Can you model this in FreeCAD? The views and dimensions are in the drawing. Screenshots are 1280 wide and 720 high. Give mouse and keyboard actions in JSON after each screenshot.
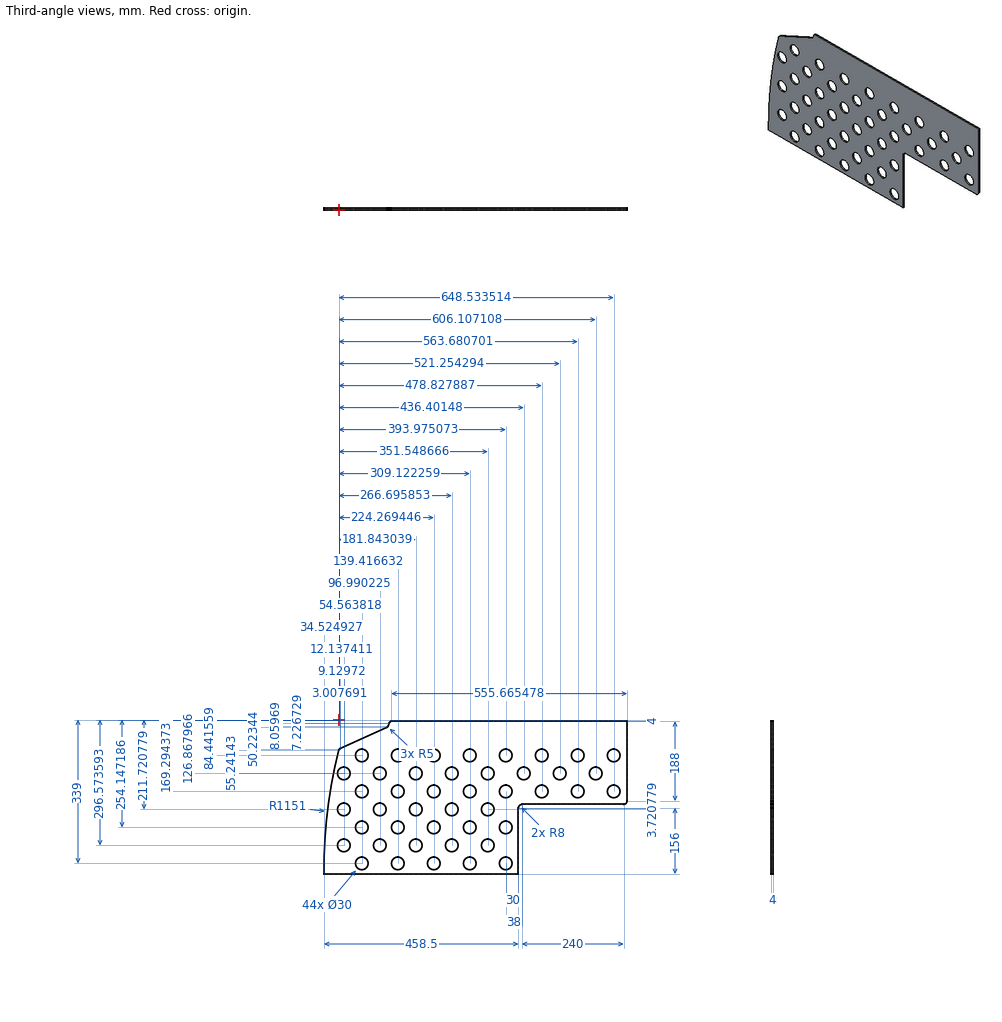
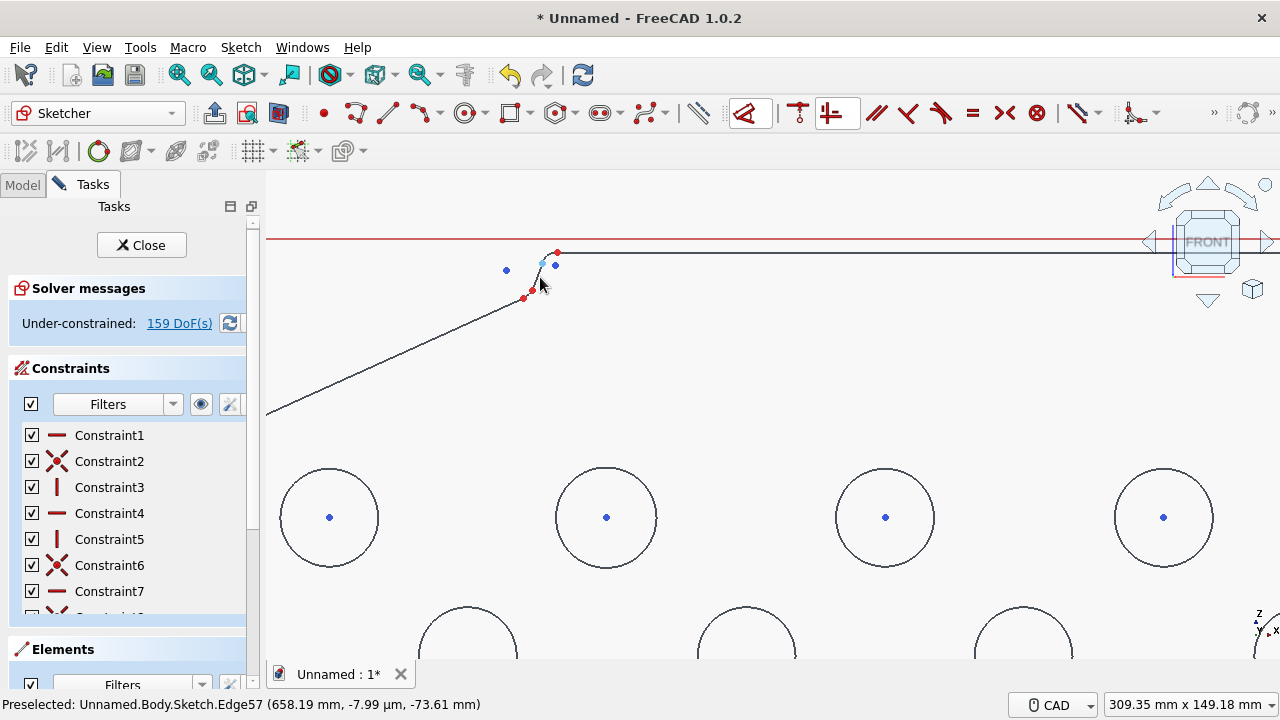
{"action": "left_click", "coordinate": [537, 277]}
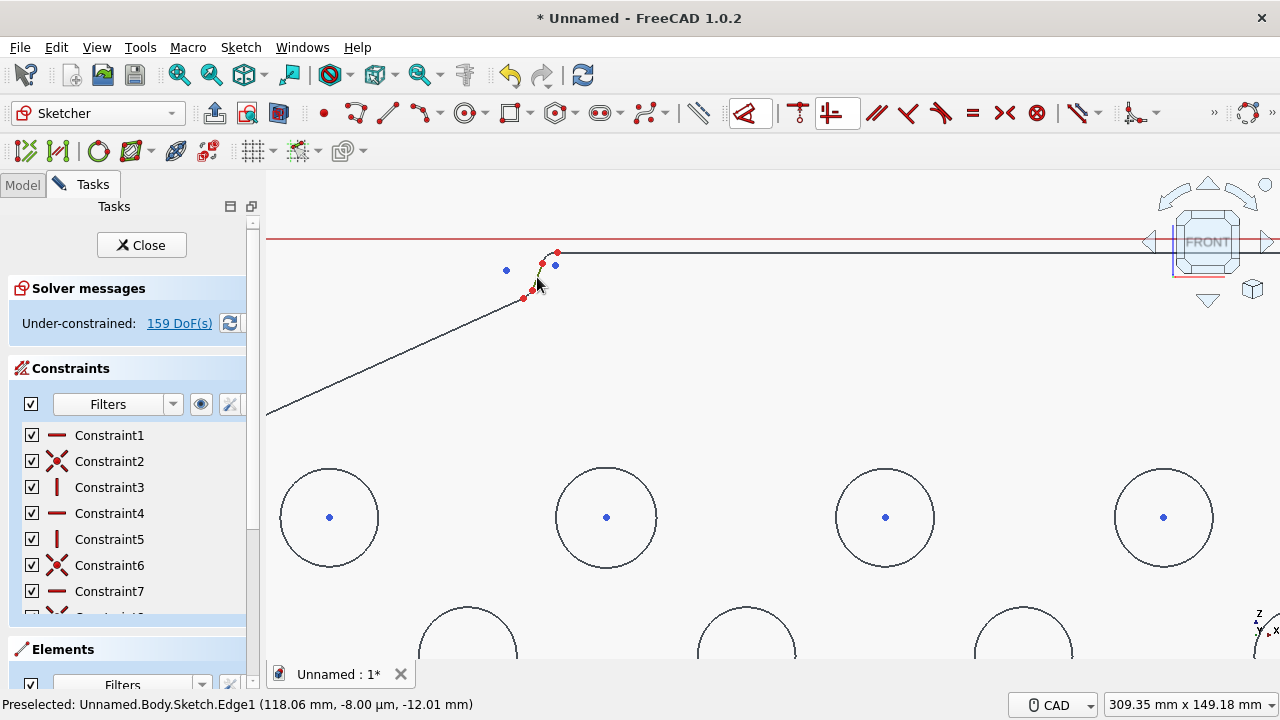
{"action": "scroll", "coordinate": [528, 295], "scroll_direction": "up", "scroll_amount": 5}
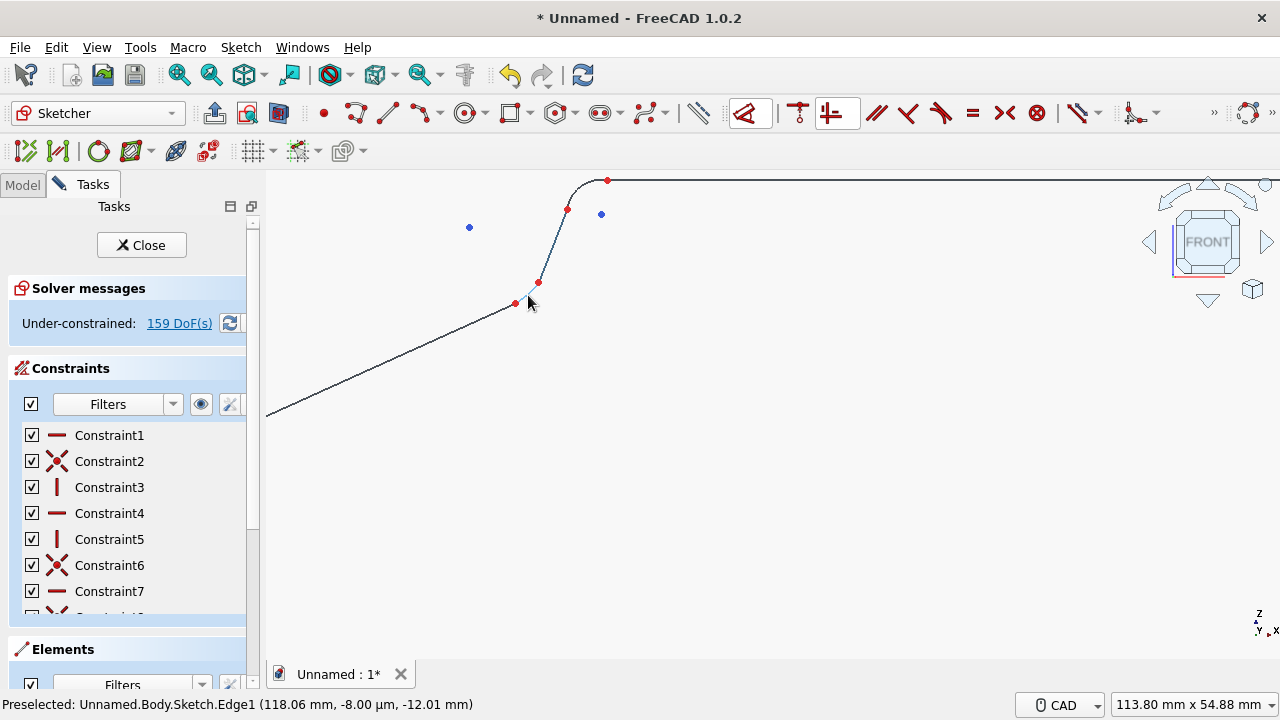
{"action": "left_click", "coordinate": [528, 294]}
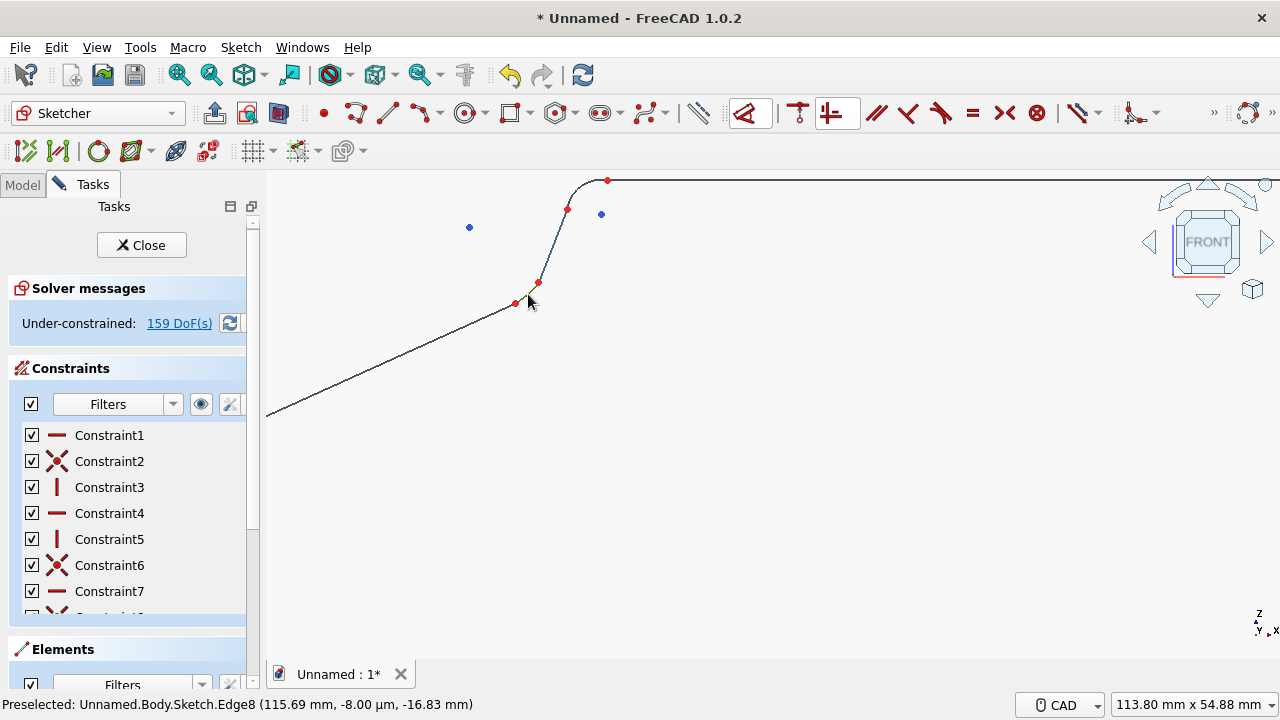
{"action": "key", "text": "t"}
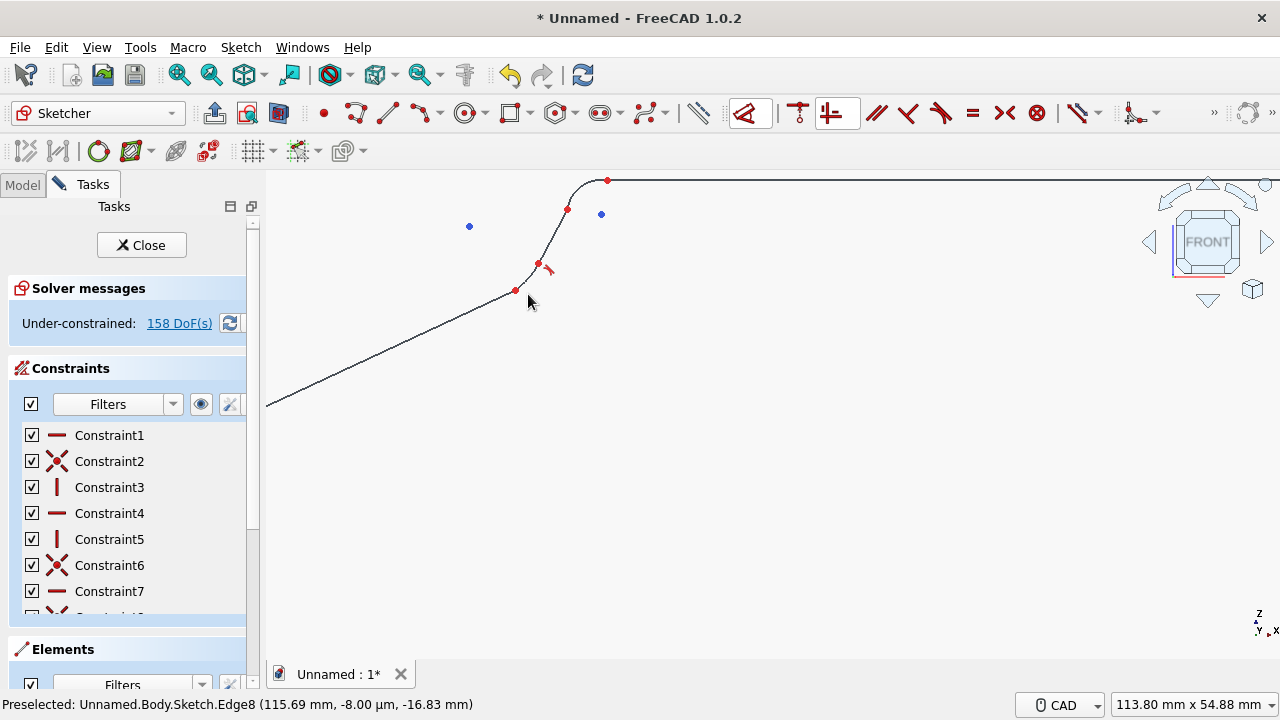
{"action": "left_click", "coordinate": [559, 226]}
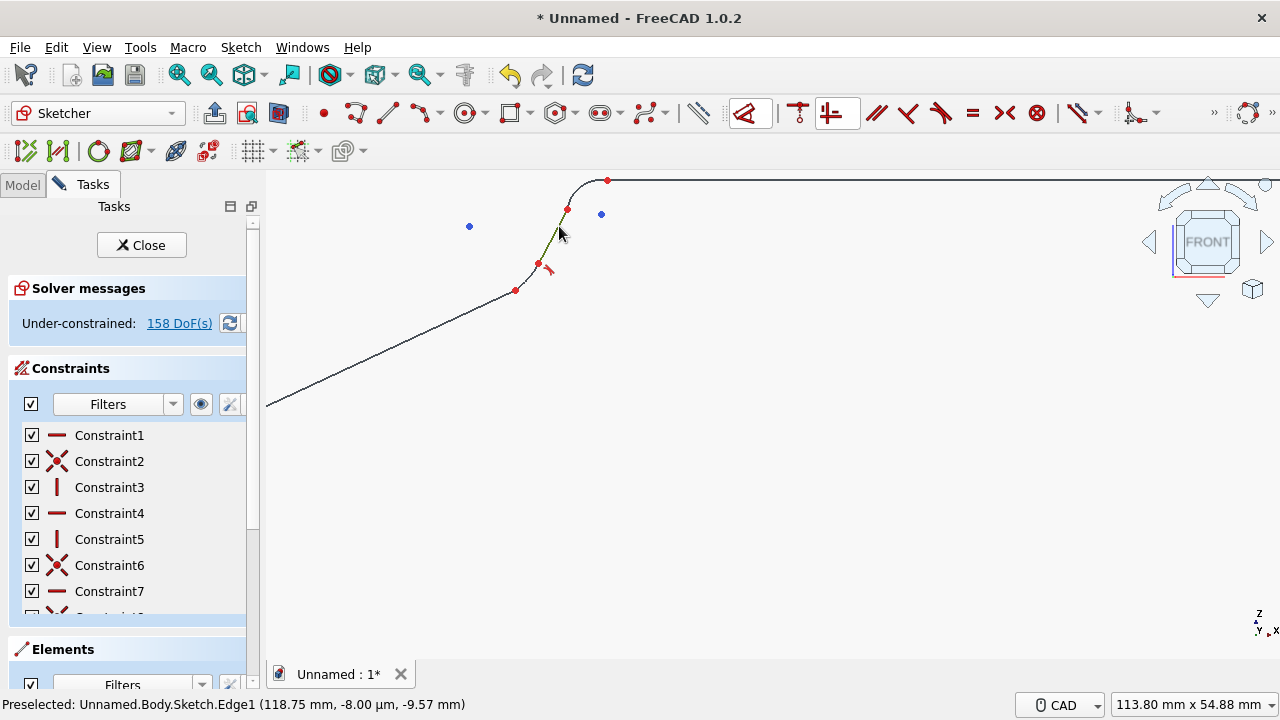
{"action": "scroll", "coordinate": [571, 199], "scroll_direction": "up", "scroll_amount": 2}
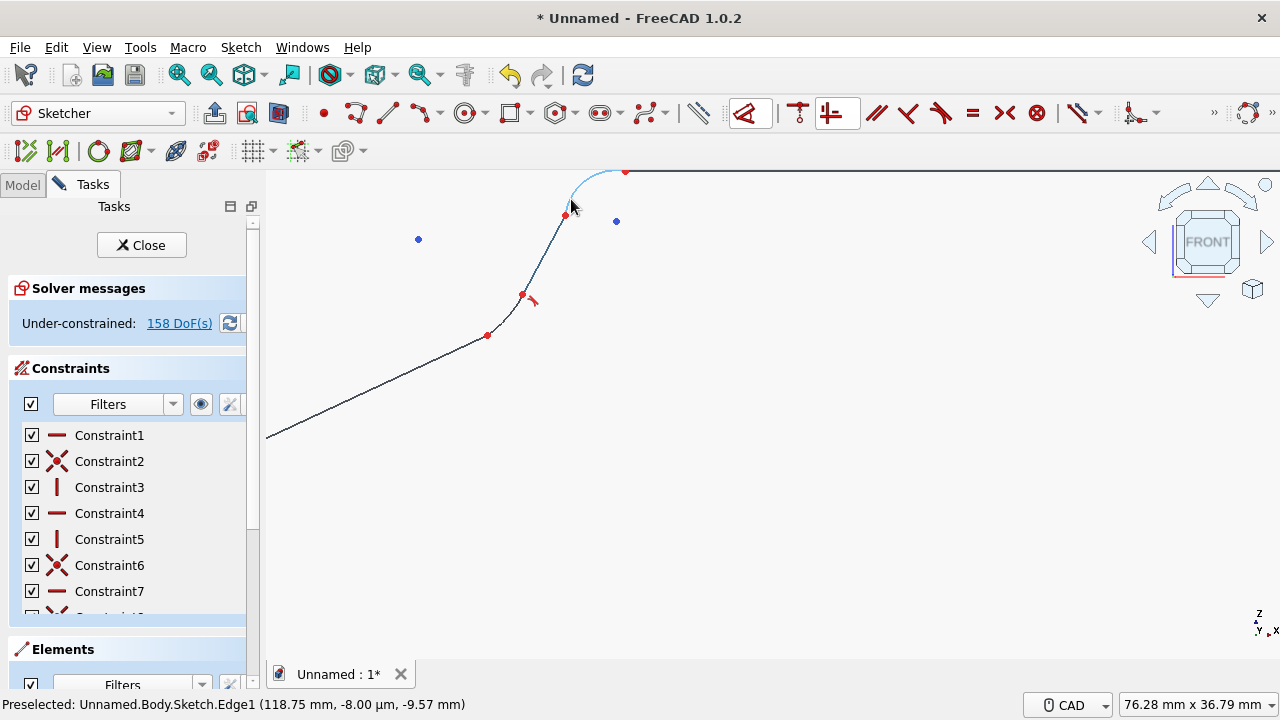
{"action": "left_click", "coordinate": [570, 199]}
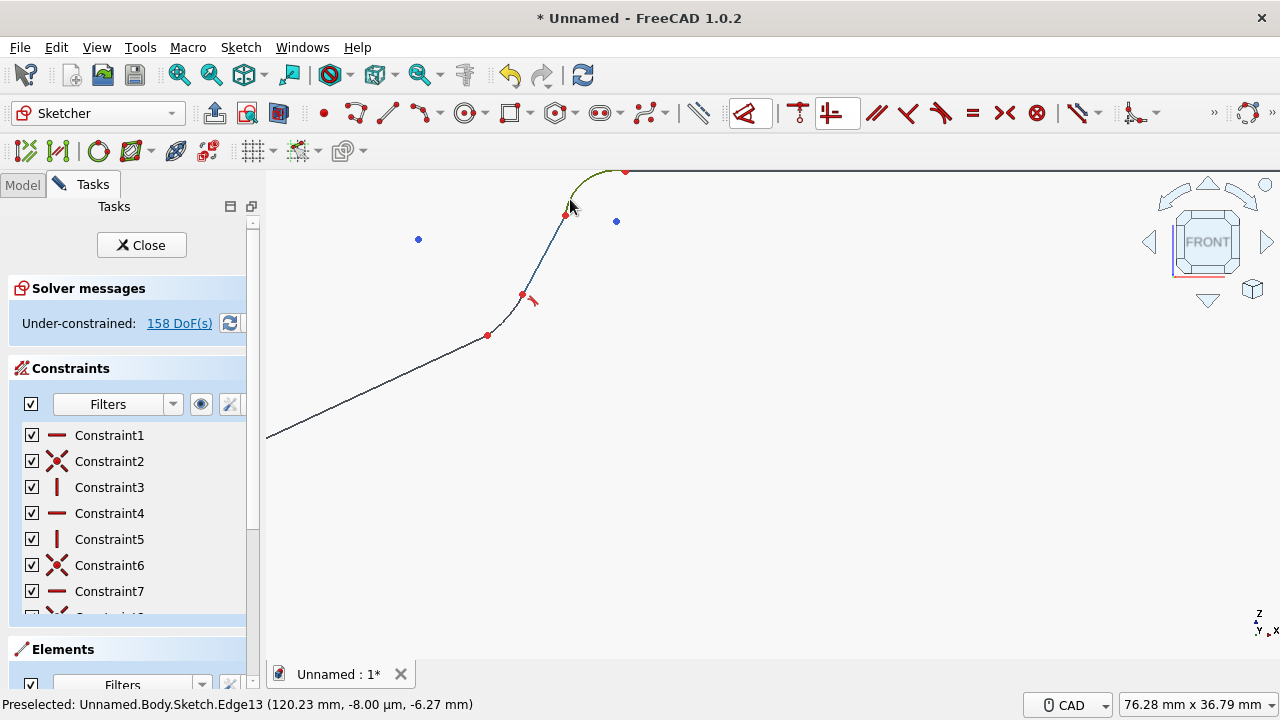
{"action": "left_click", "coordinate": [942, 114]}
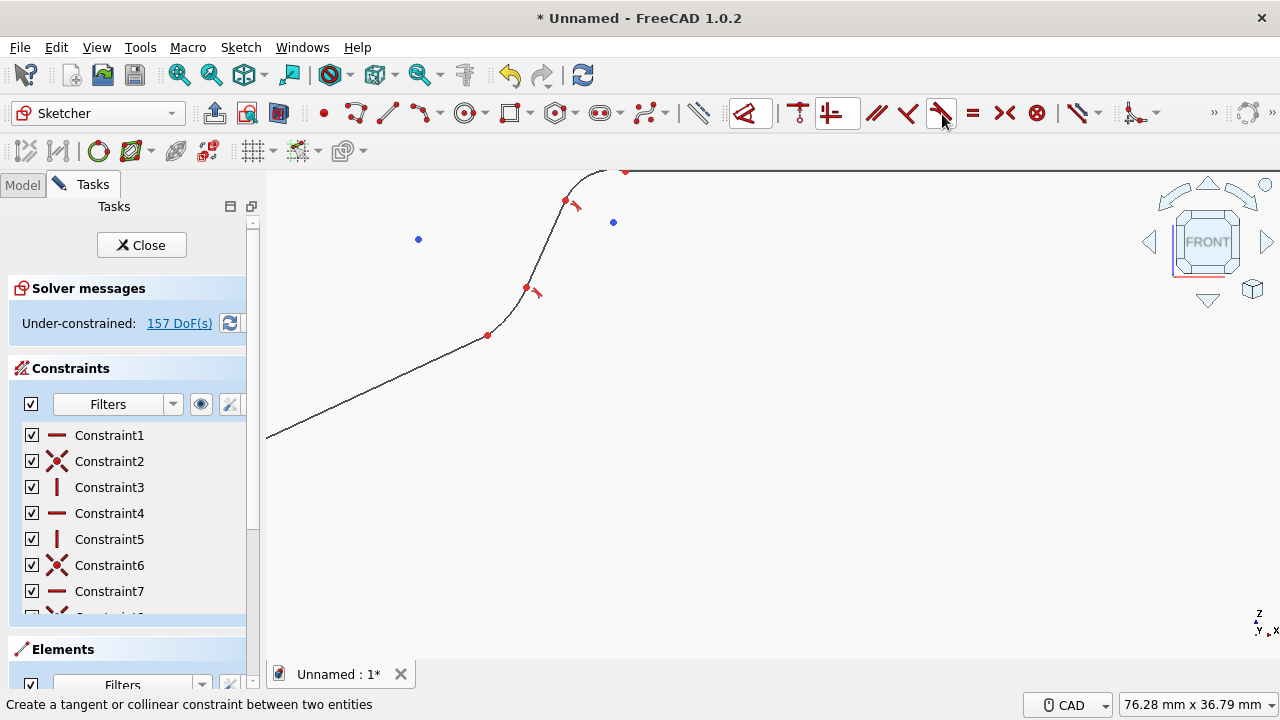
{"action": "scroll", "coordinate": [539, 277], "scroll_direction": "down", "scroll_amount": 14}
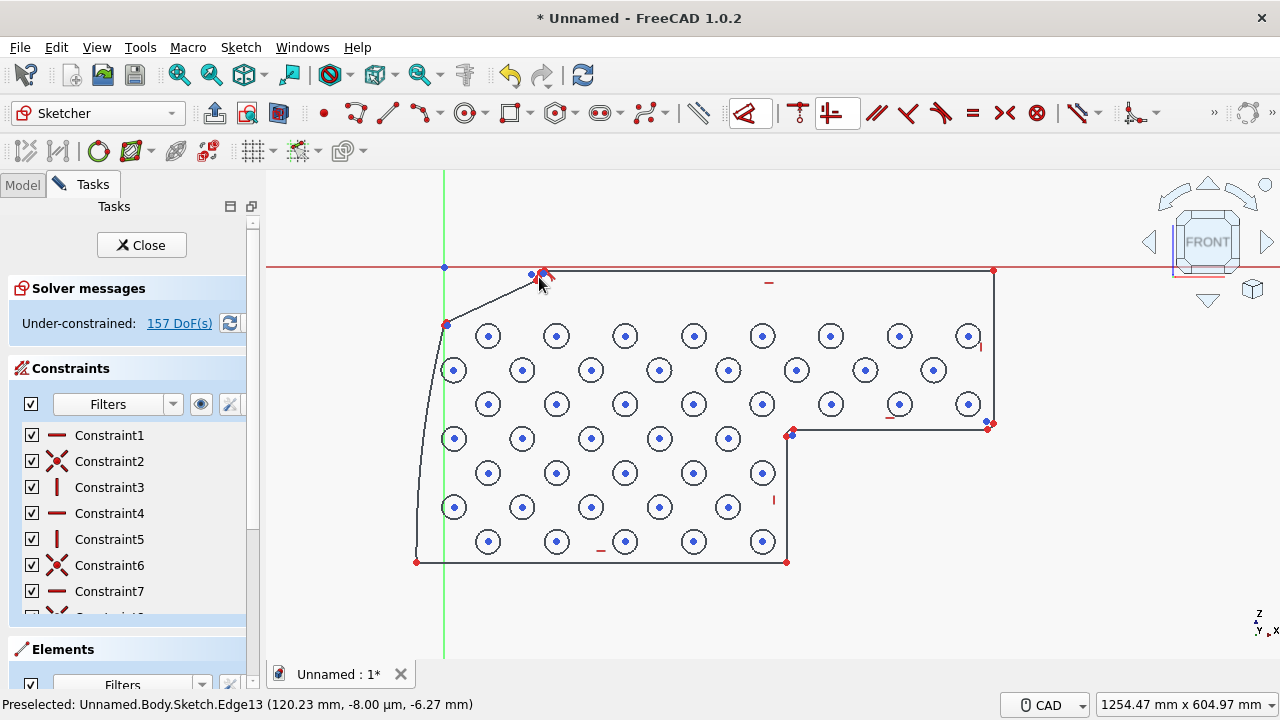
{"action": "left_click", "coordinate": [509, 293]}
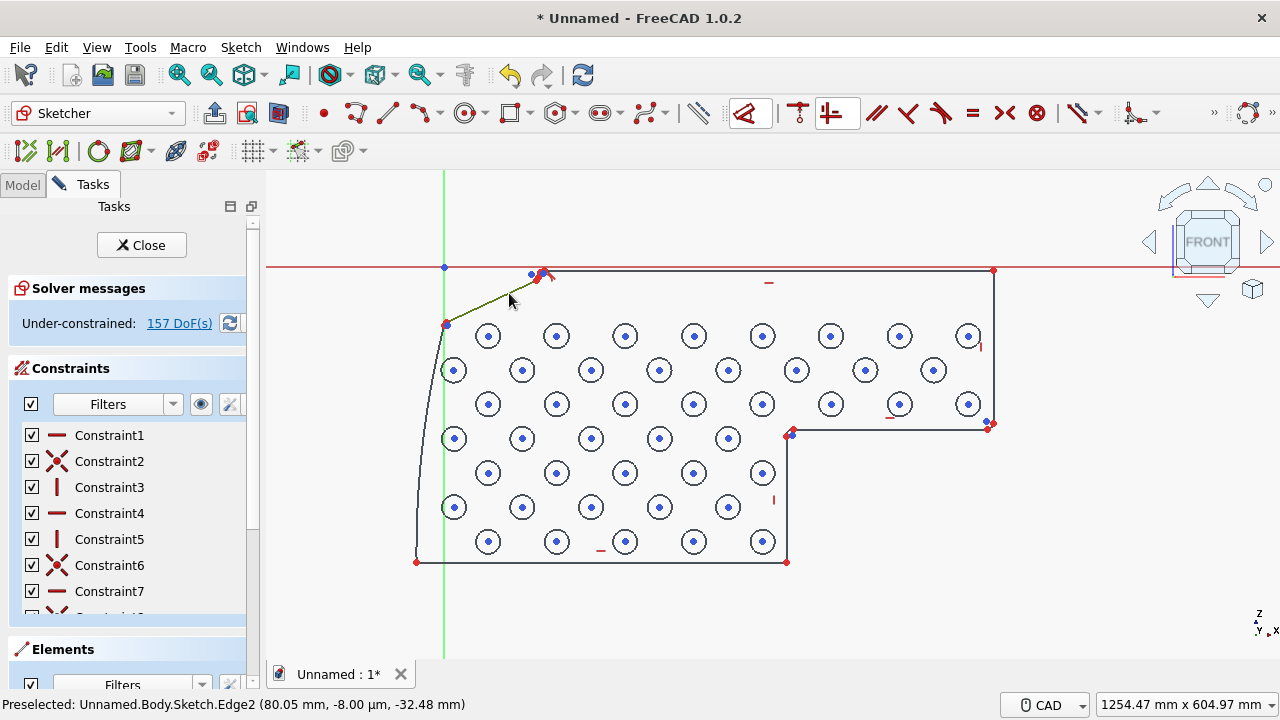
{"action": "scroll", "coordinate": [538, 279], "scroll_direction": "up", "scroll_amount": 10}